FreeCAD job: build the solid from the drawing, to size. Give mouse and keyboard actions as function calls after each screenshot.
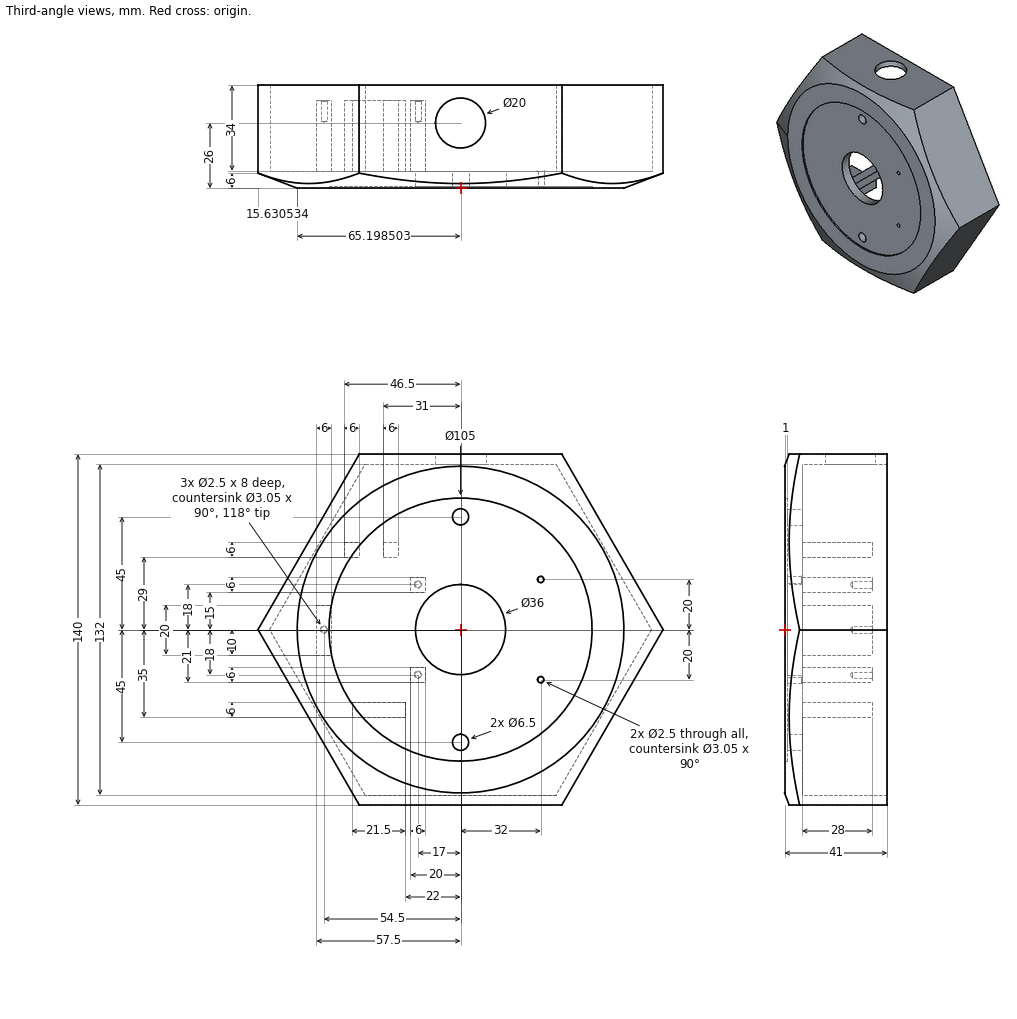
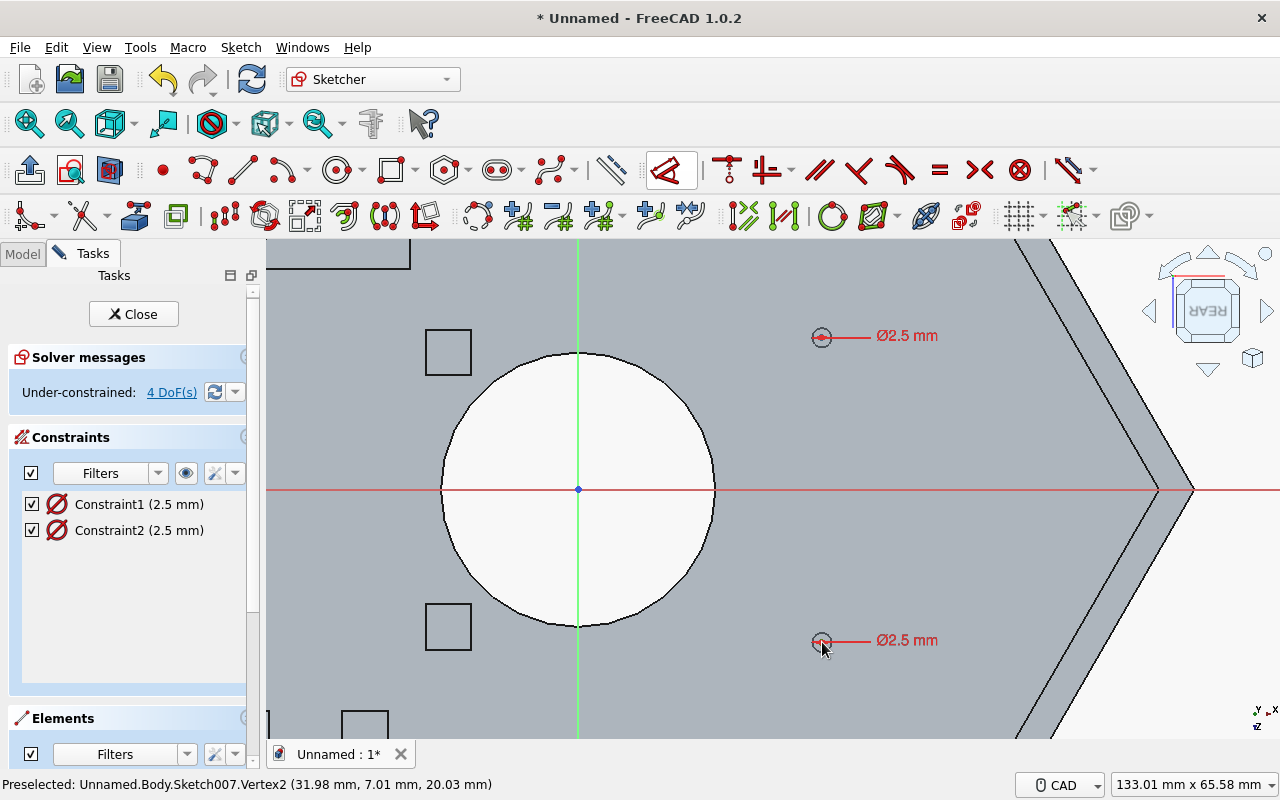
key(v)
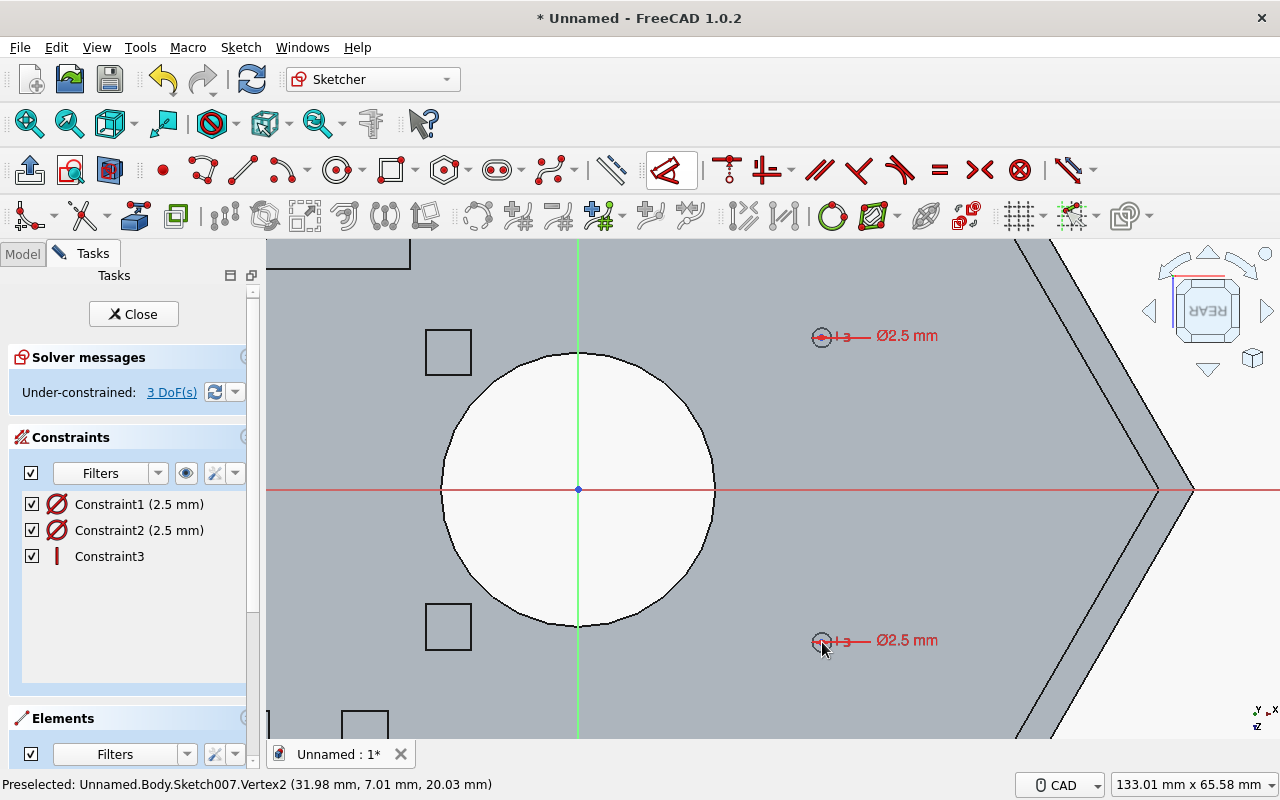
click(822, 338)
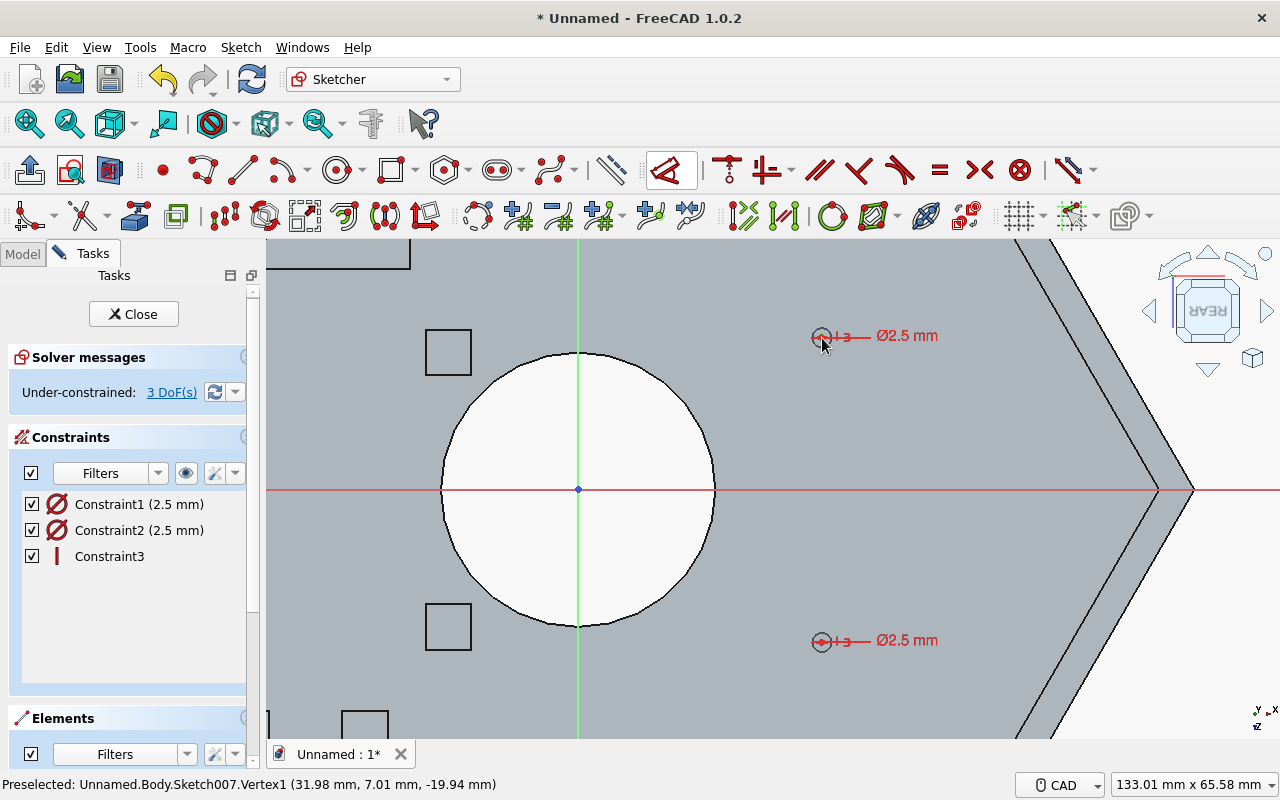
key(l)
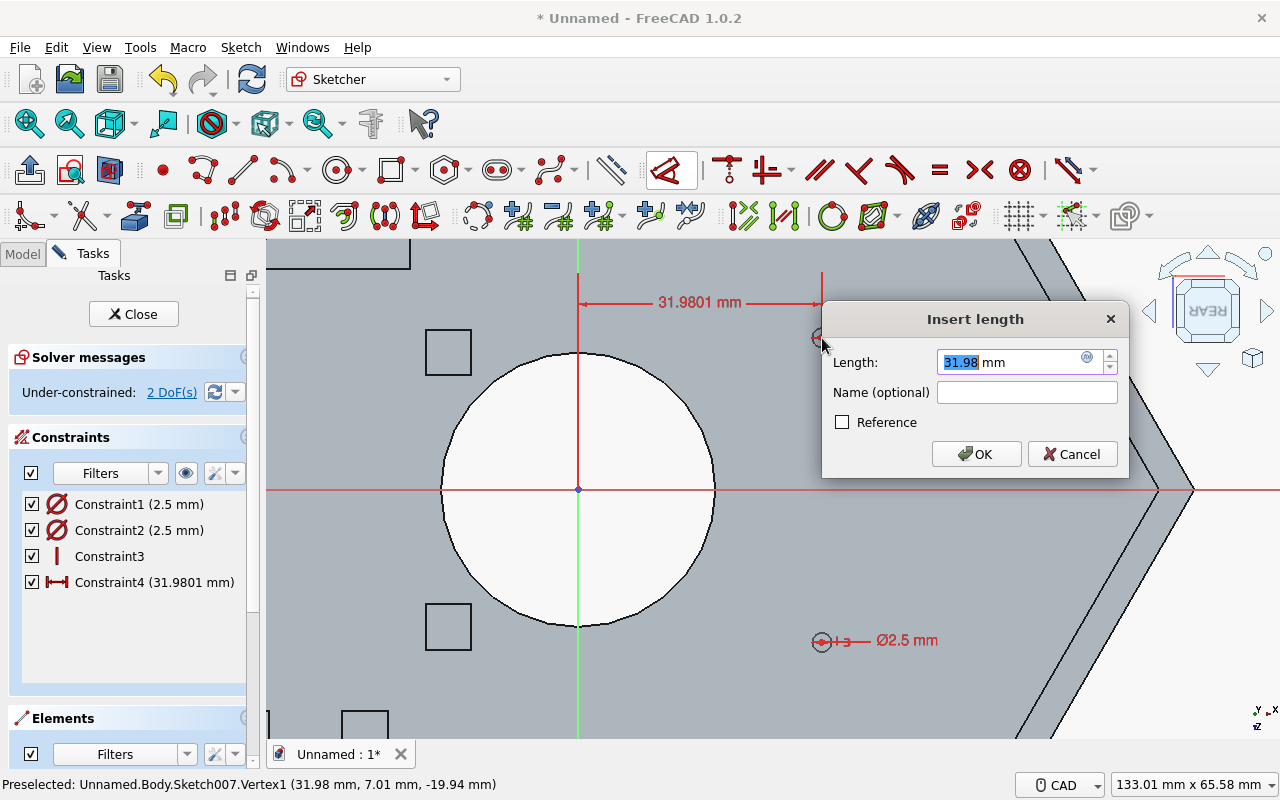
text(32)
key(Return)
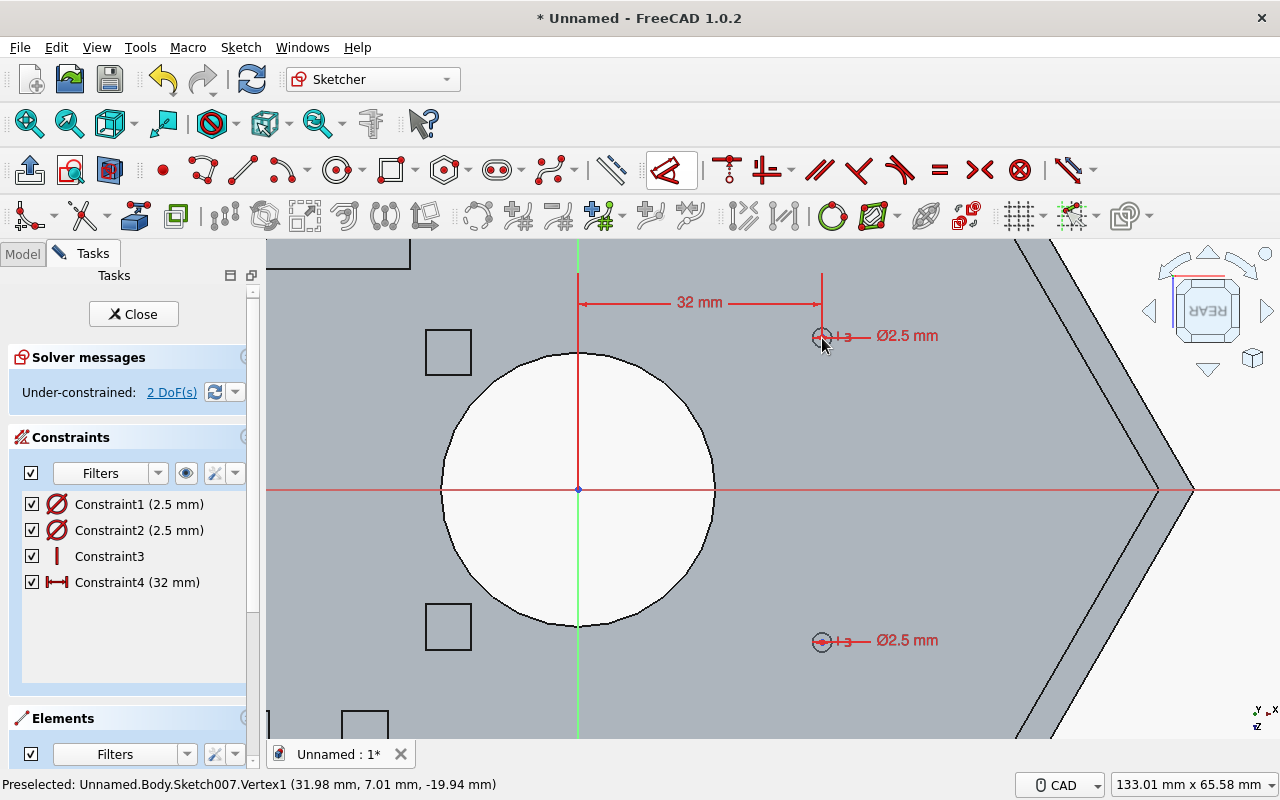
click(822, 338)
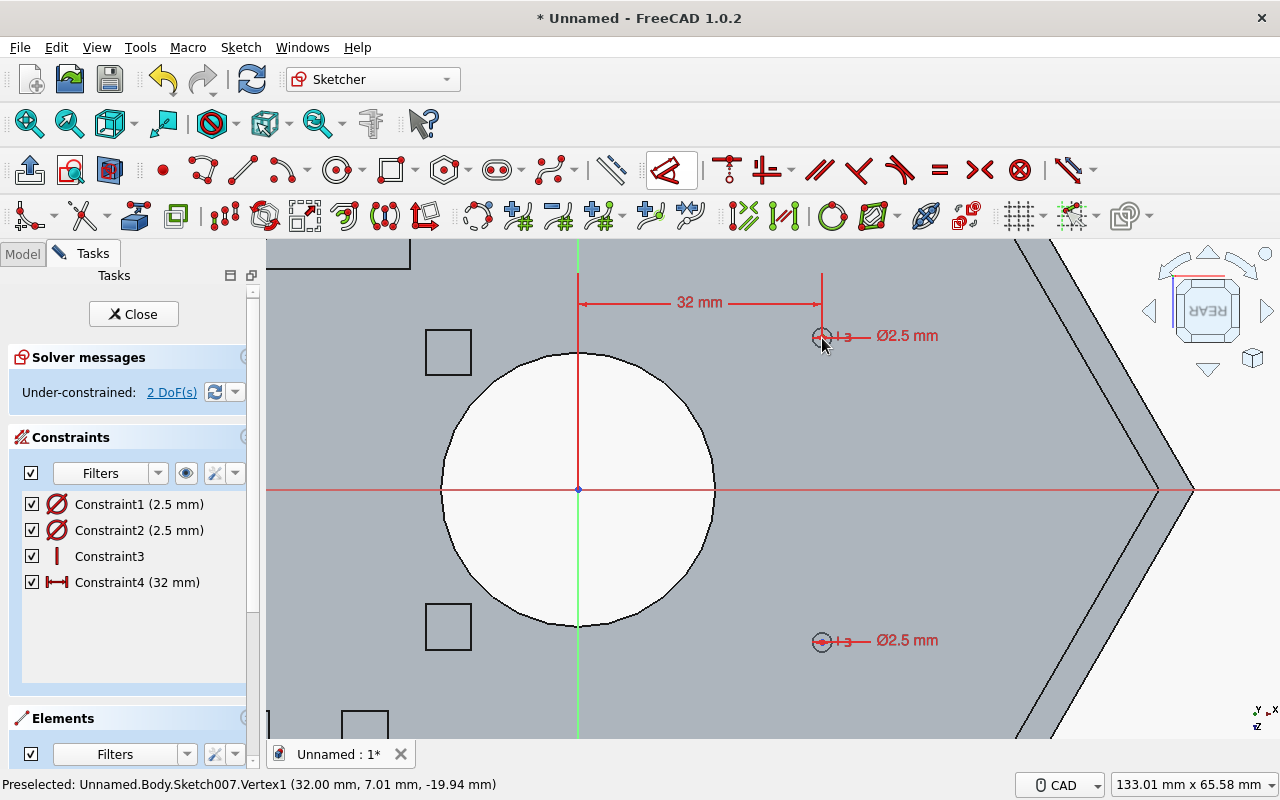
key(i)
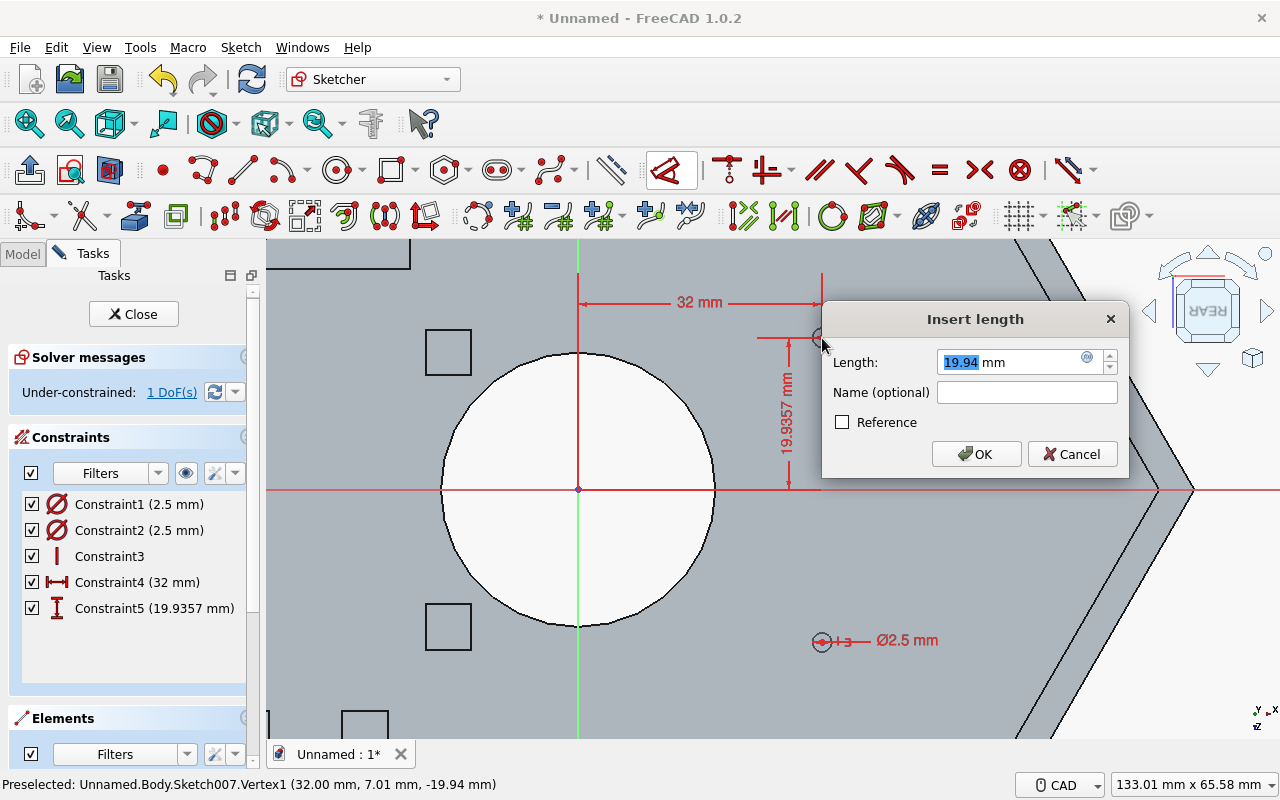
text(20)
key(Return)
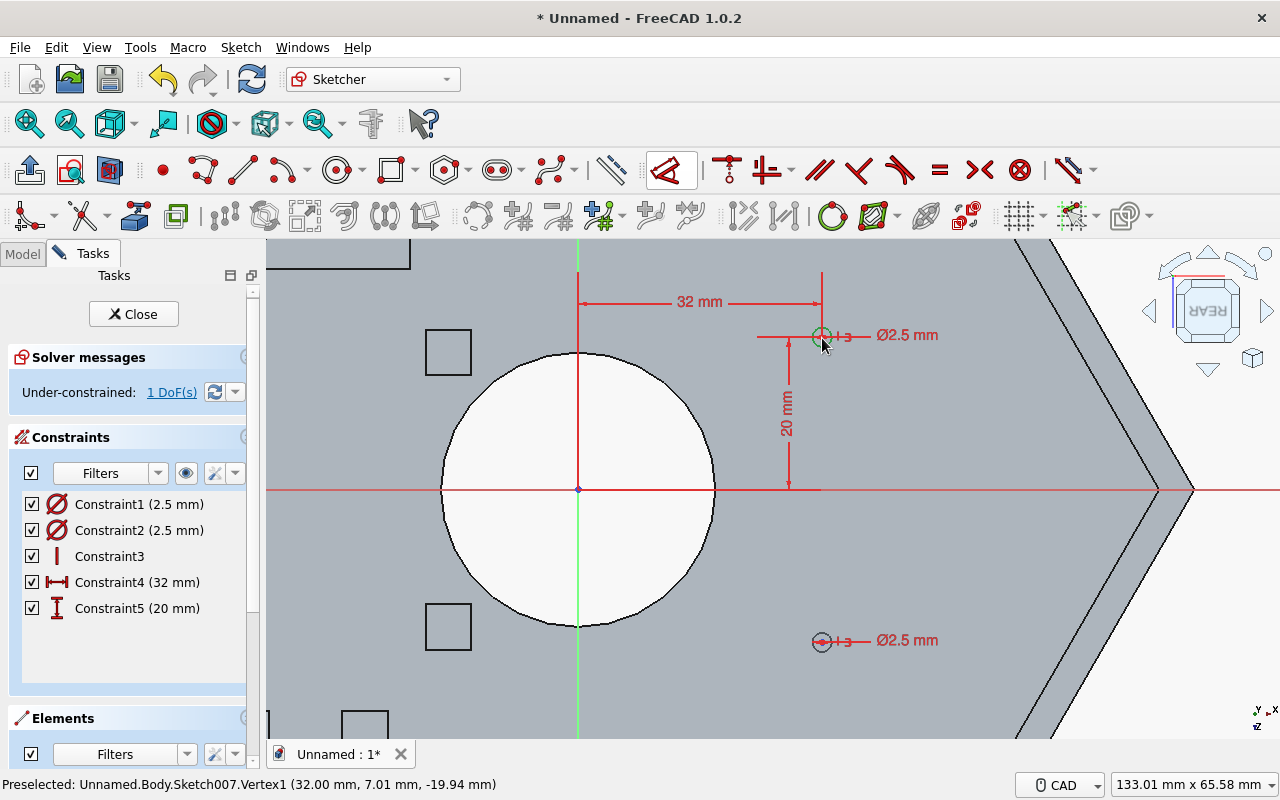
click(822, 642)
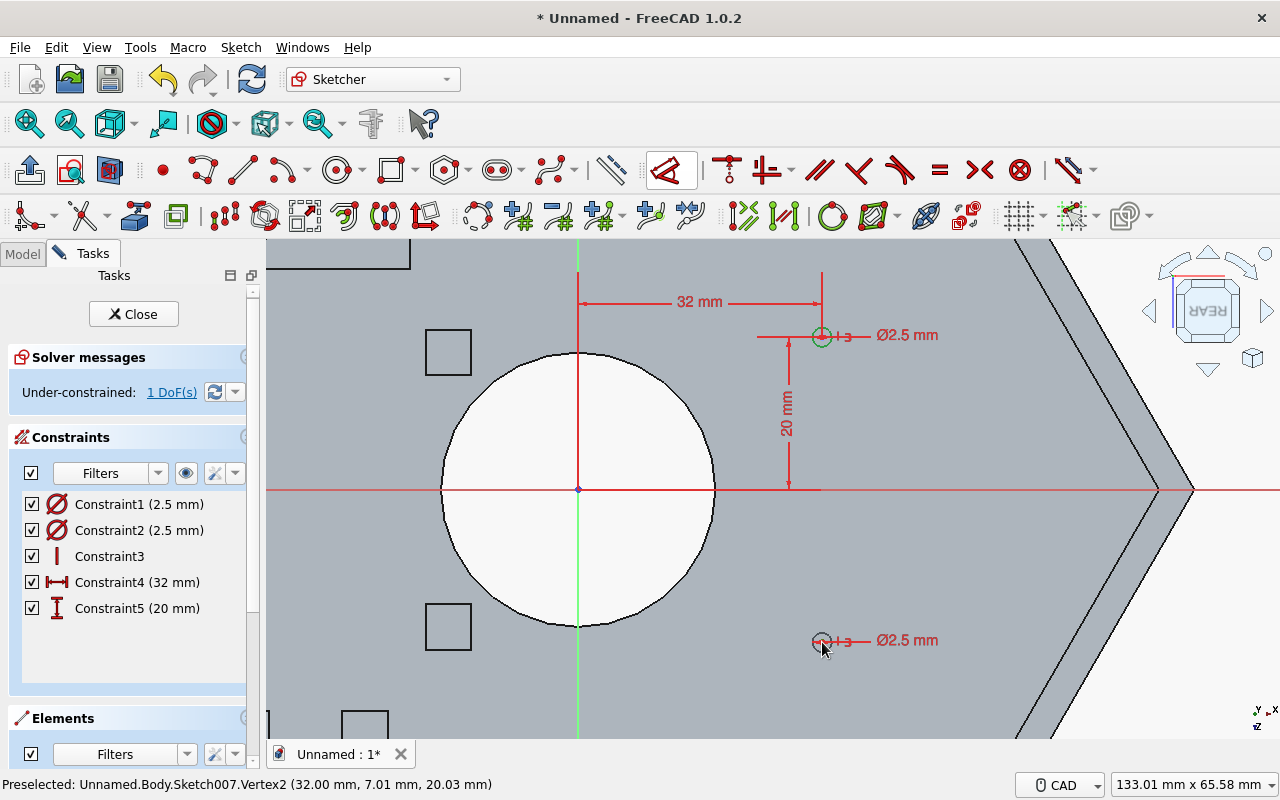
click(692, 170)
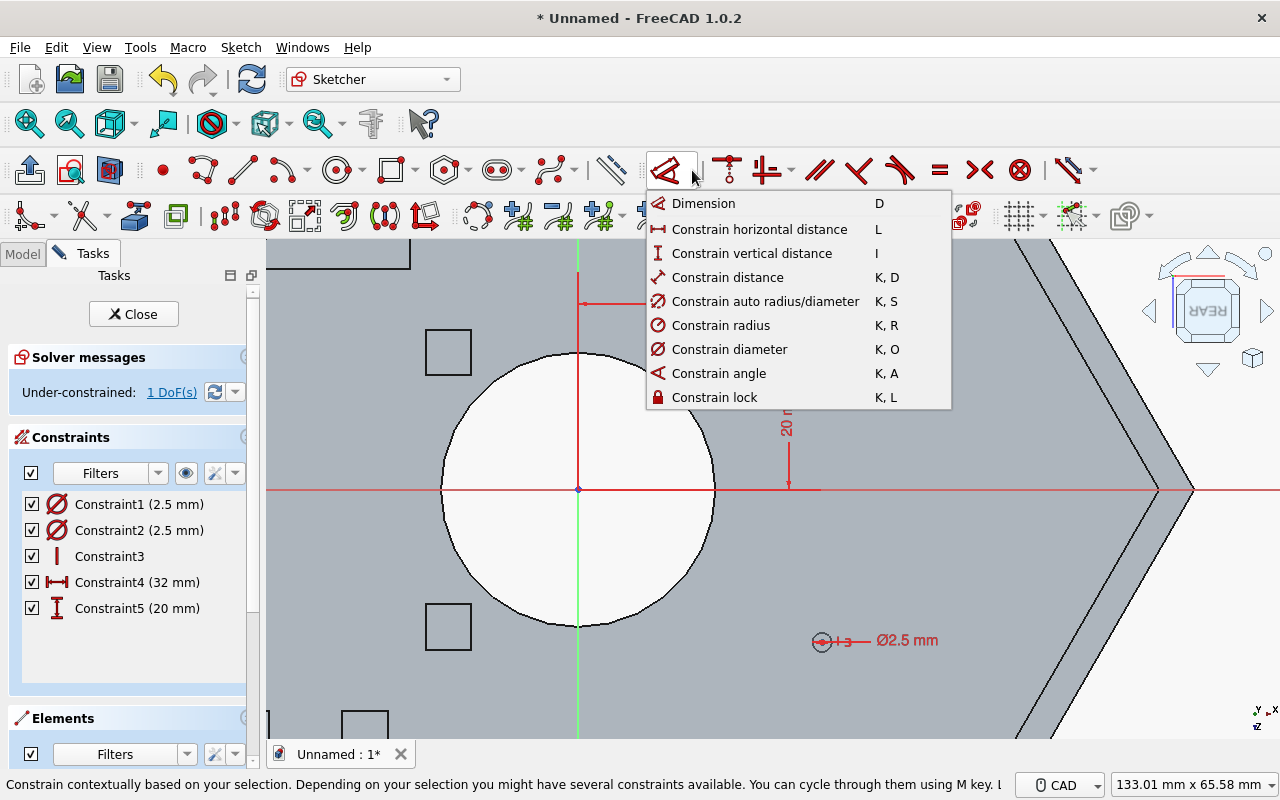
click(799, 253)